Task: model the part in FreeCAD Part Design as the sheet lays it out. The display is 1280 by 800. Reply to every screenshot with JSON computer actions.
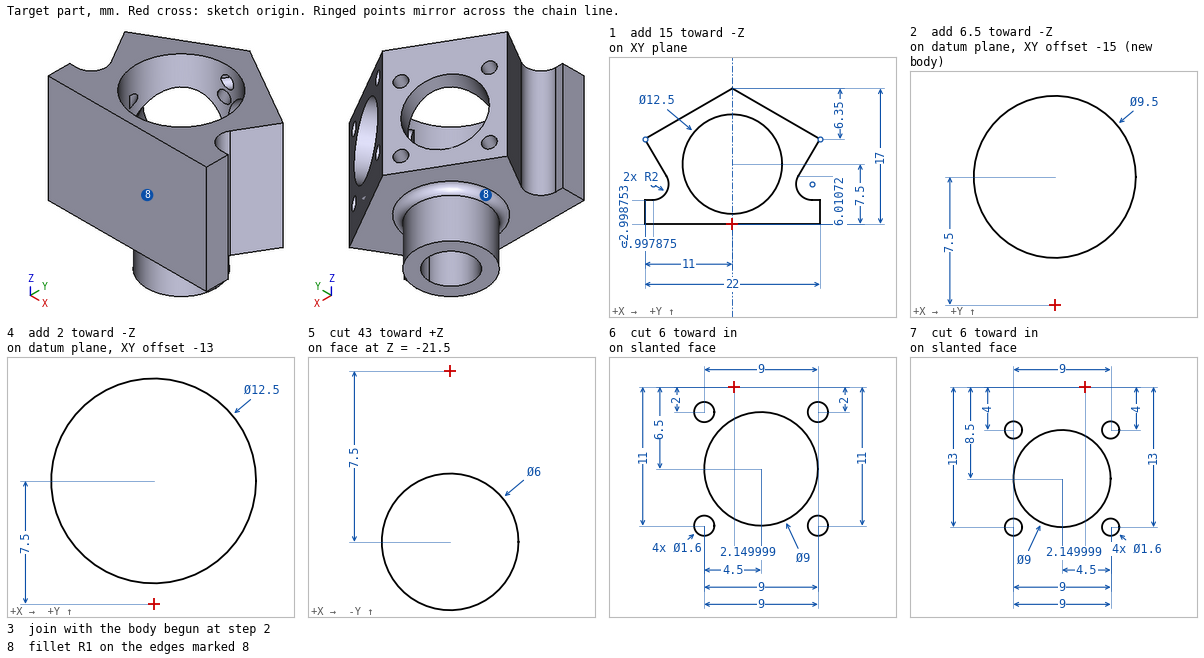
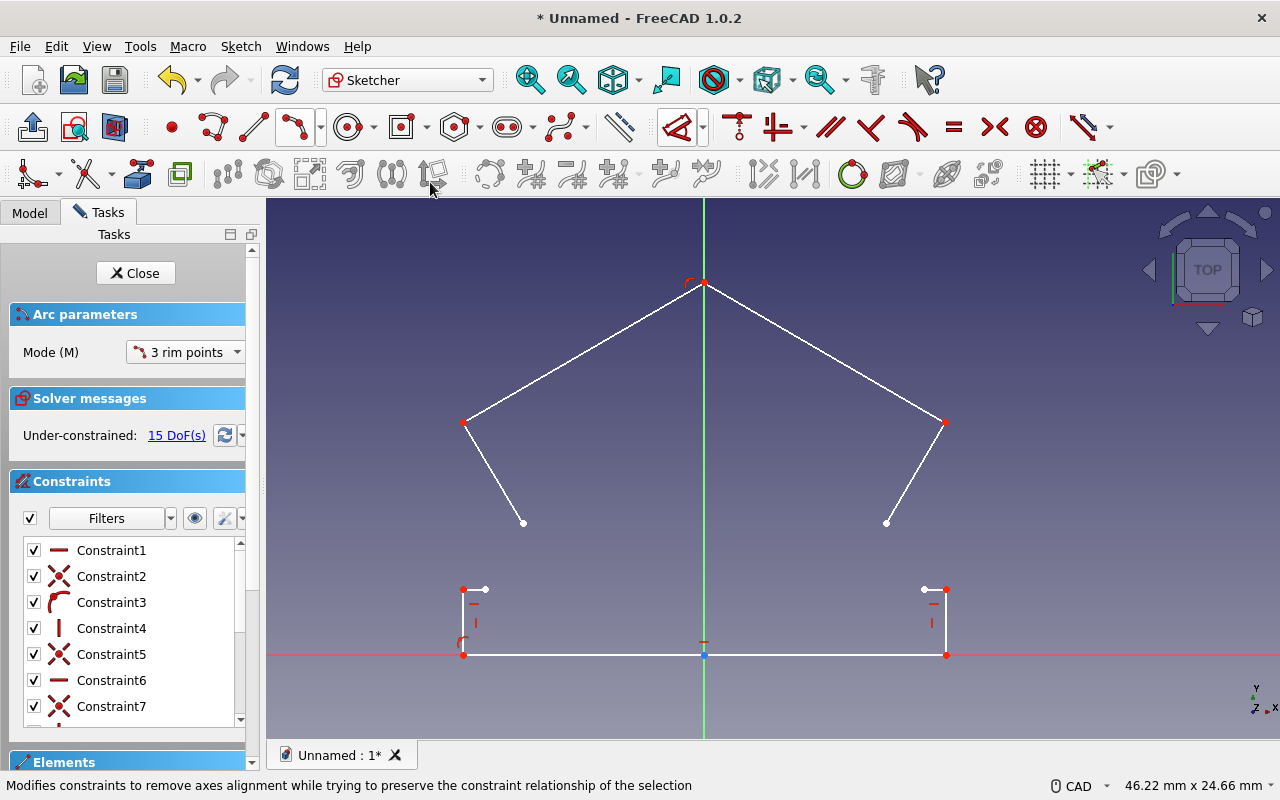
{"action": "scroll", "coordinate": [924, 589], "scroll_direction": "up", "scroll_amount": 2}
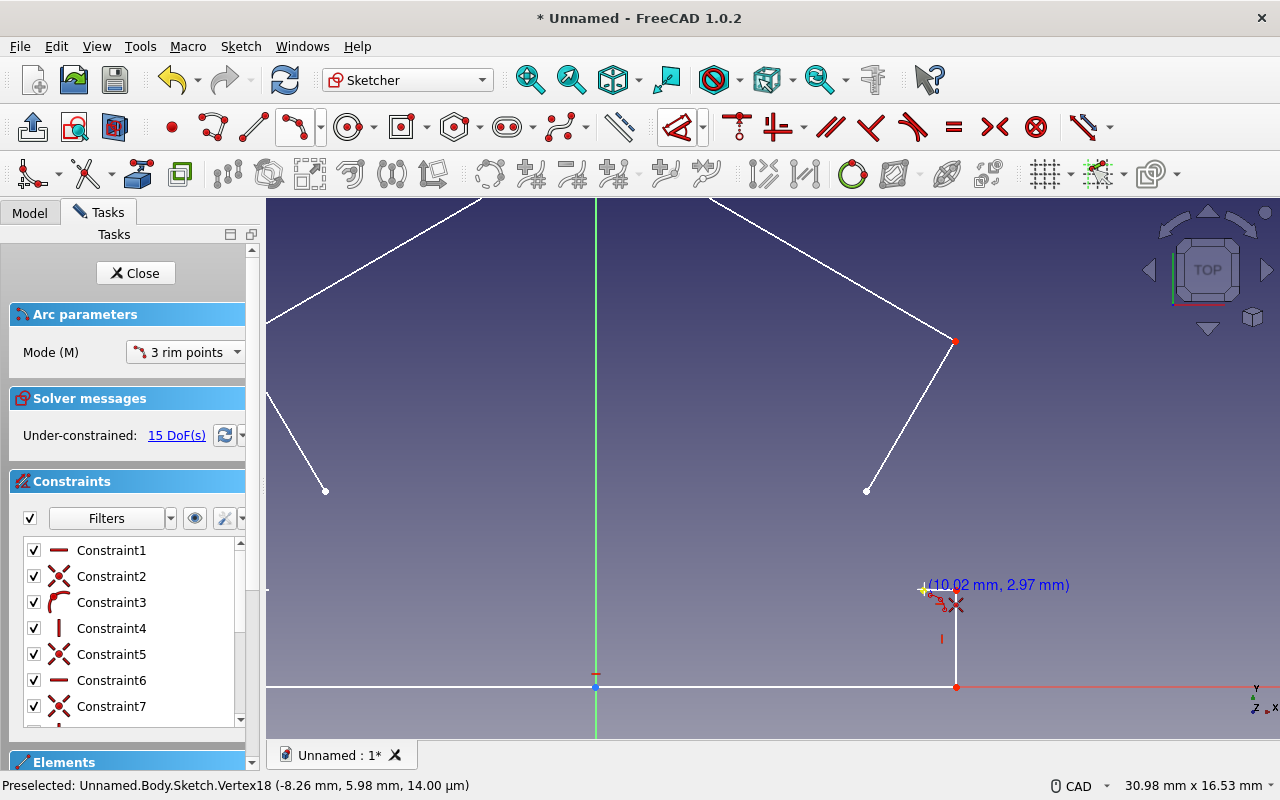
{"action": "left_click", "coordinate": [924, 590]}
{"action": "left_click", "coordinate": [867, 492]}
{"action": "left_click", "coordinate": [866, 556]}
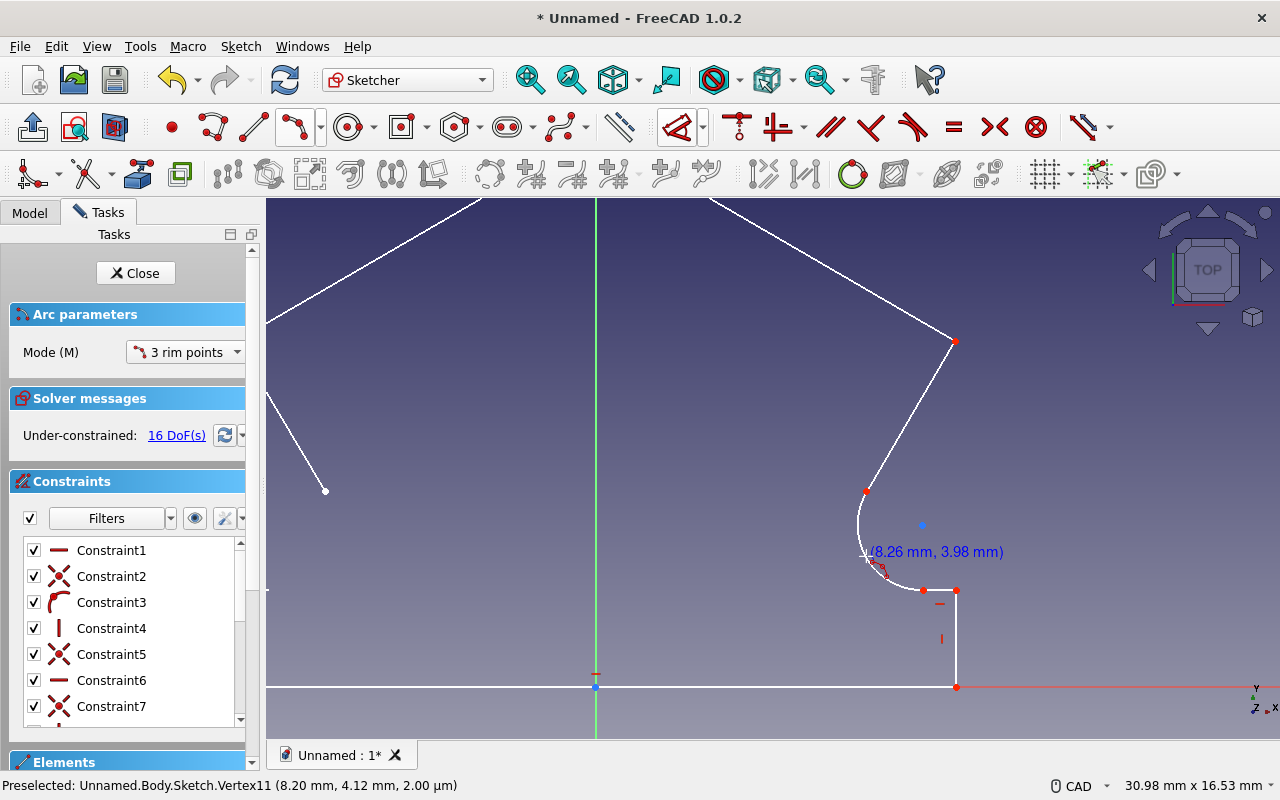
{"action": "left_click", "coordinate": [325, 492]}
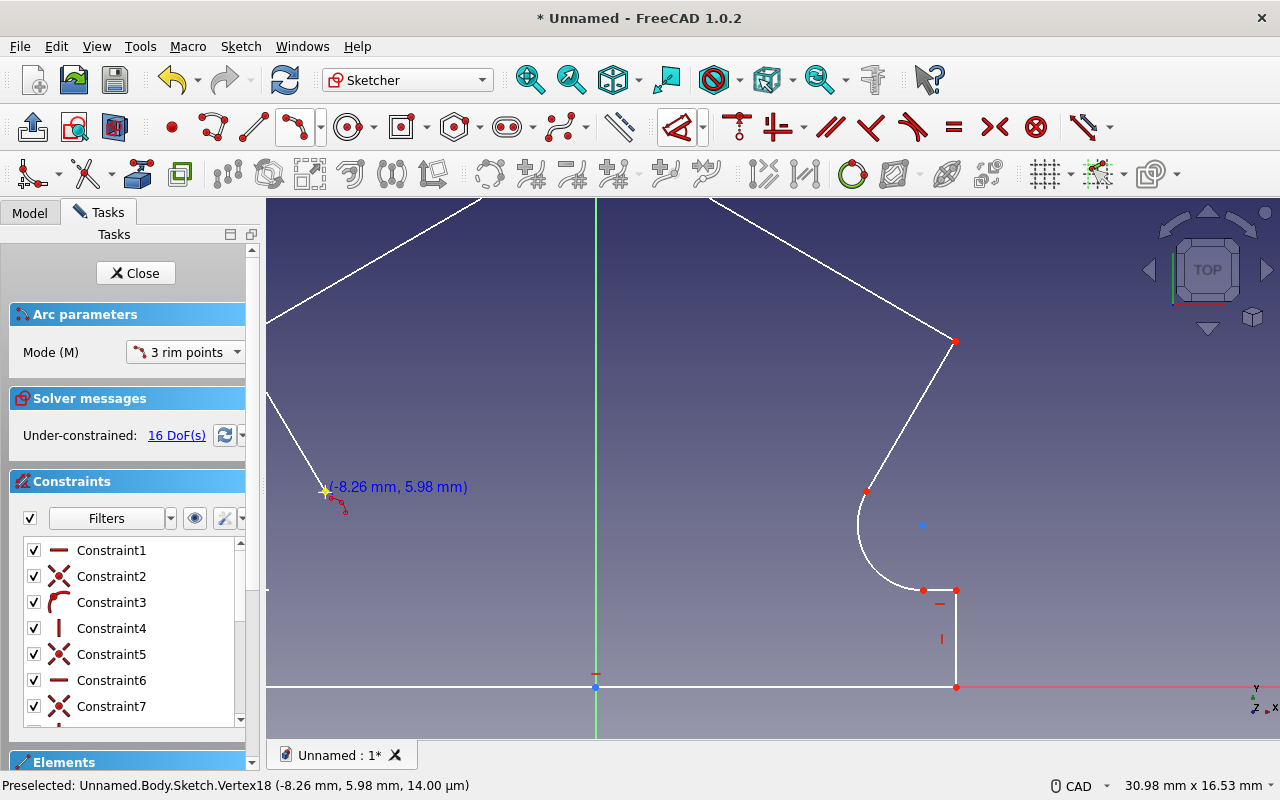
{"action": "scroll", "coordinate": [926, 589], "scroll_direction": "down", "scroll_amount": 2}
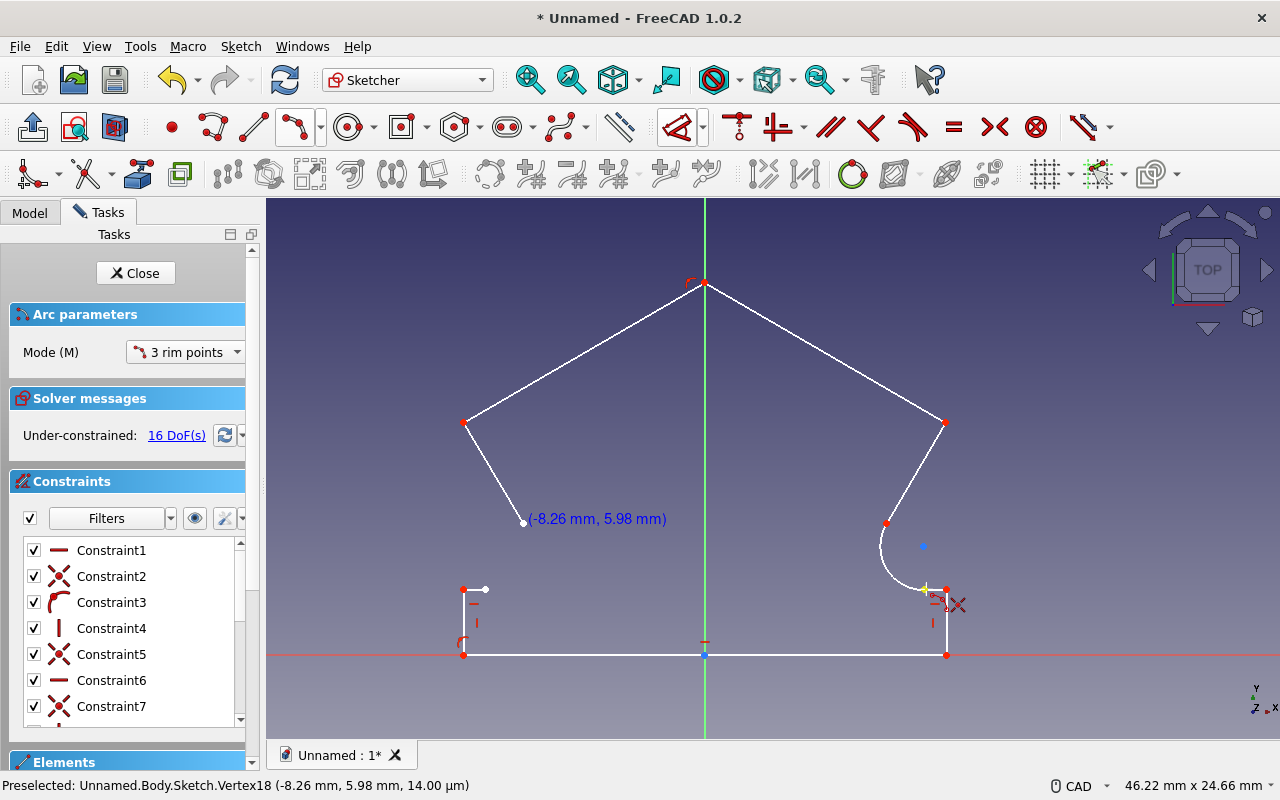
{"action": "scroll", "coordinate": [485, 589], "scroll_direction": "up", "scroll_amount": 2}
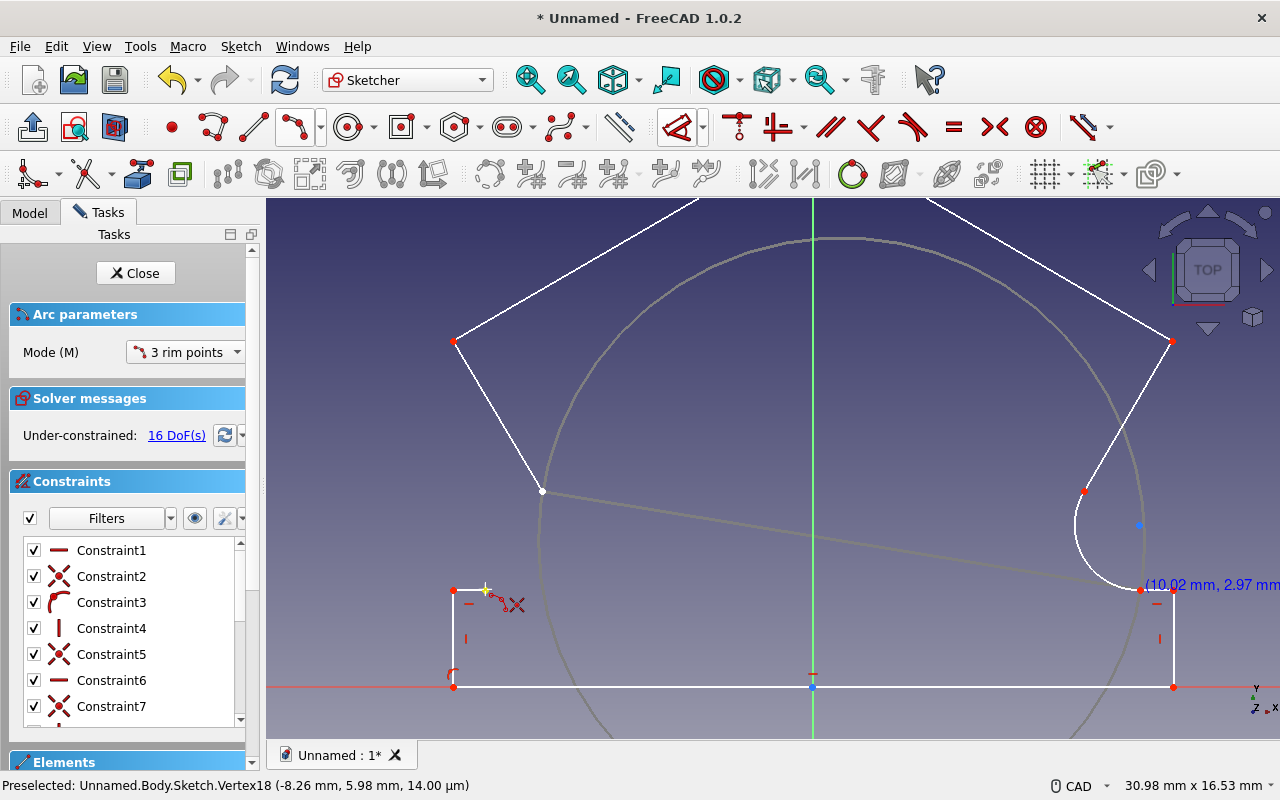
{"action": "left_click", "coordinate": [486, 590]}
{"action": "left_click", "coordinate": [542, 556]}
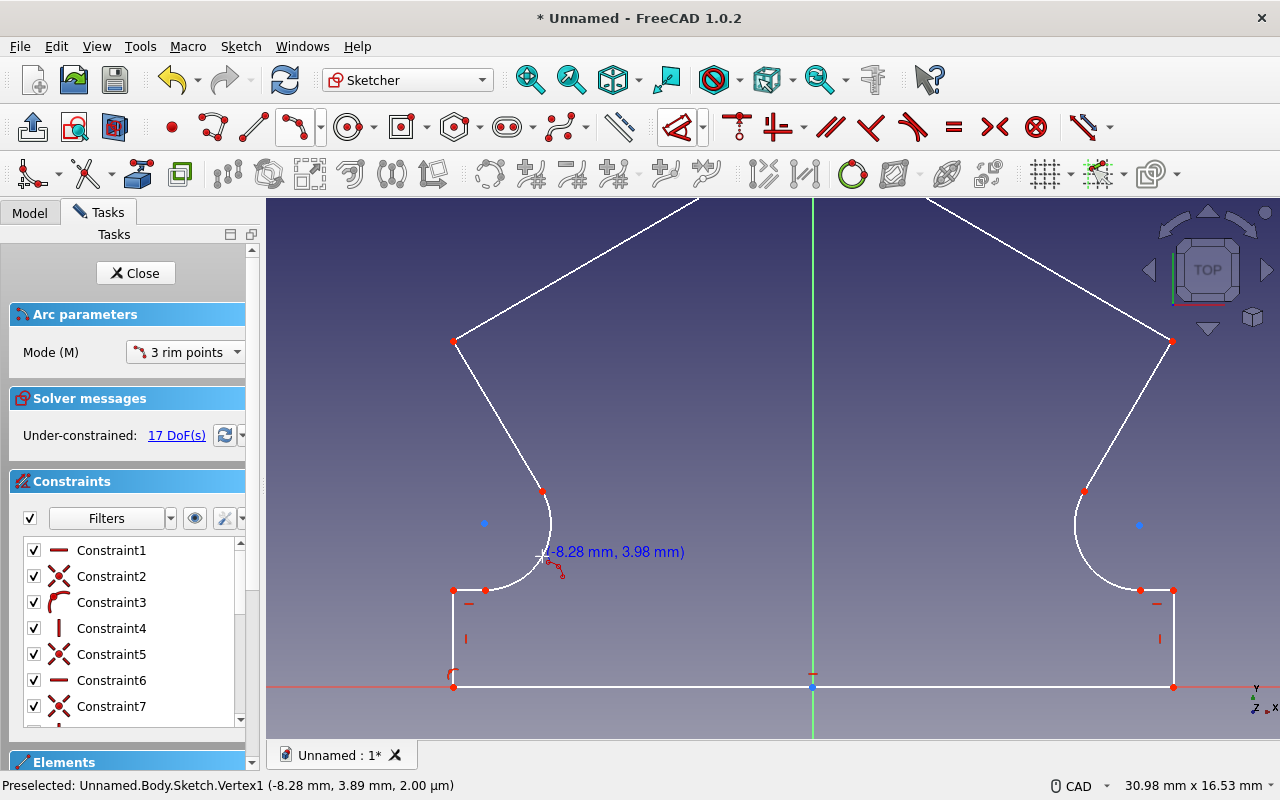
{"action": "left_click", "coordinate": [348, 128]}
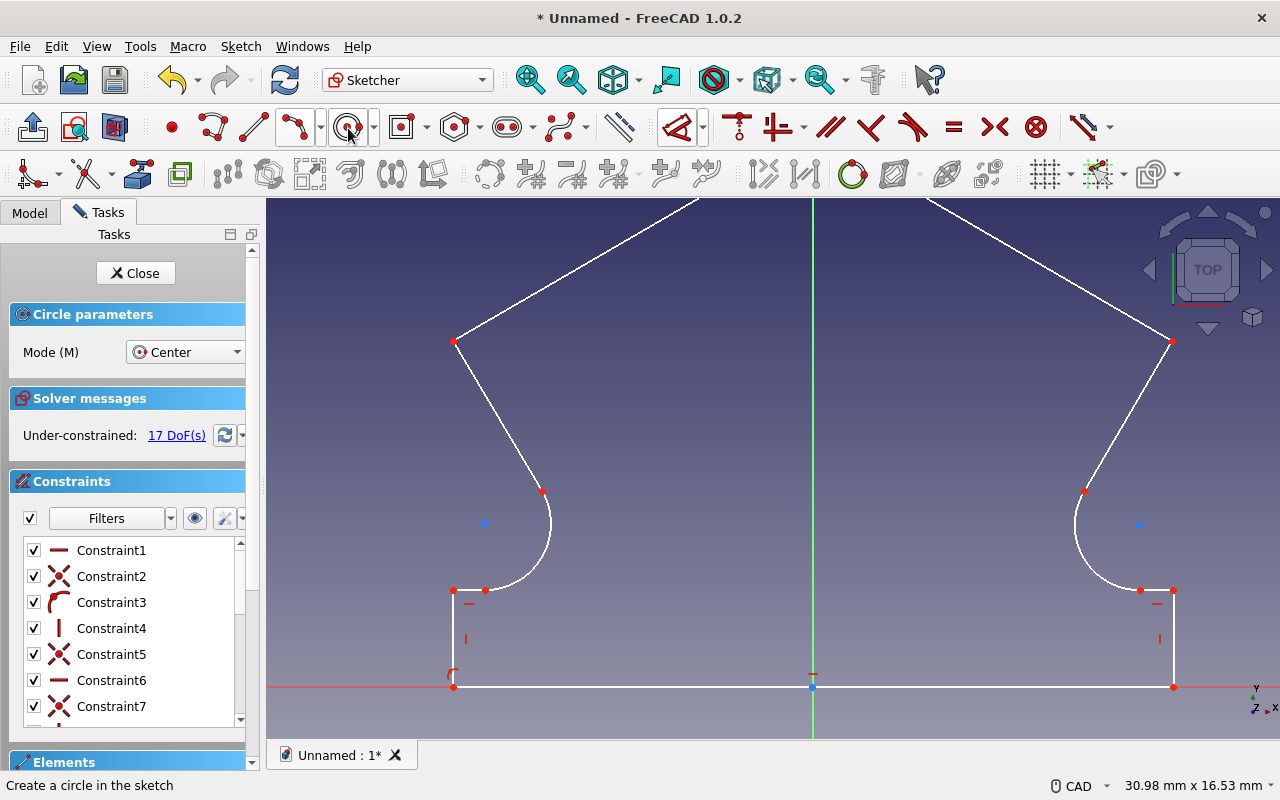
{"action": "left_click", "coordinate": [813, 442]}
{"action": "mouse_move", "coordinate": [958, 297]}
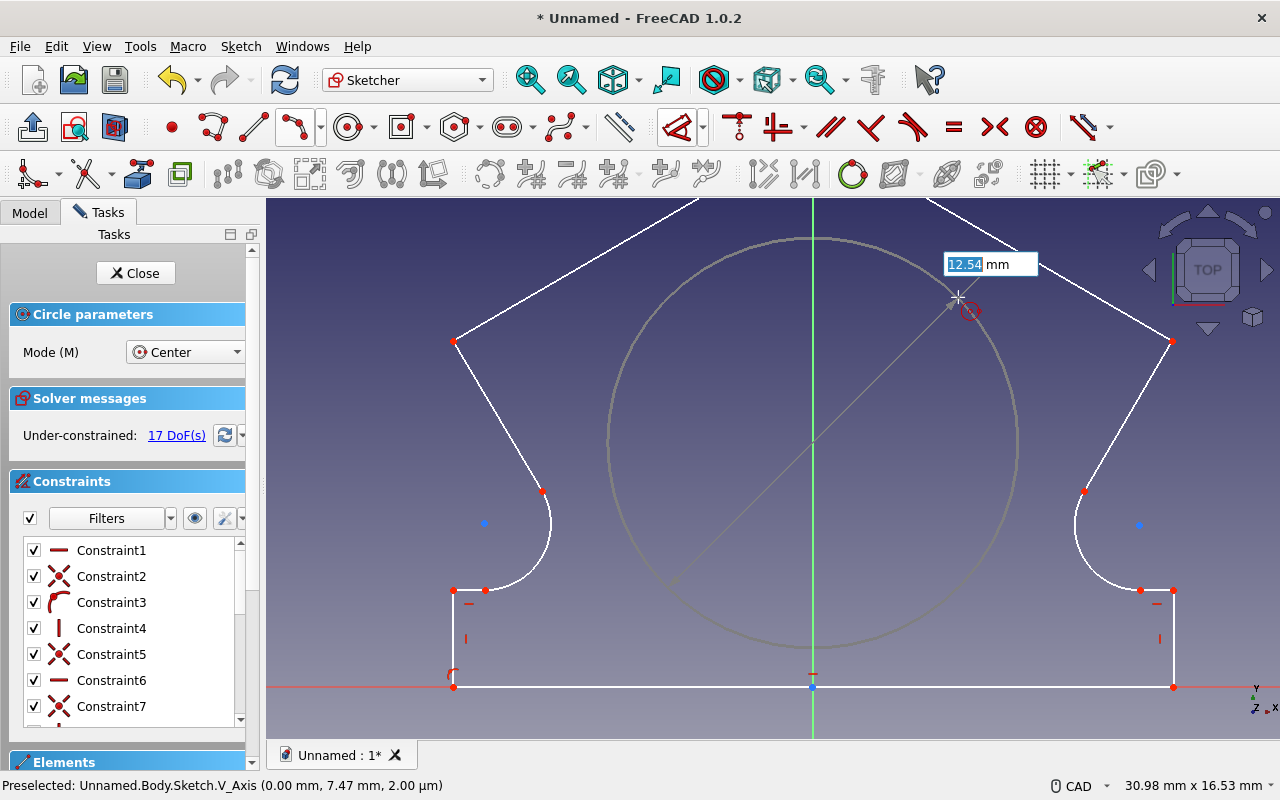
{"action": "type", "text": "12.5"}
{"action": "key", "text": "Return"}
{"action": "key", "text": "Escape"}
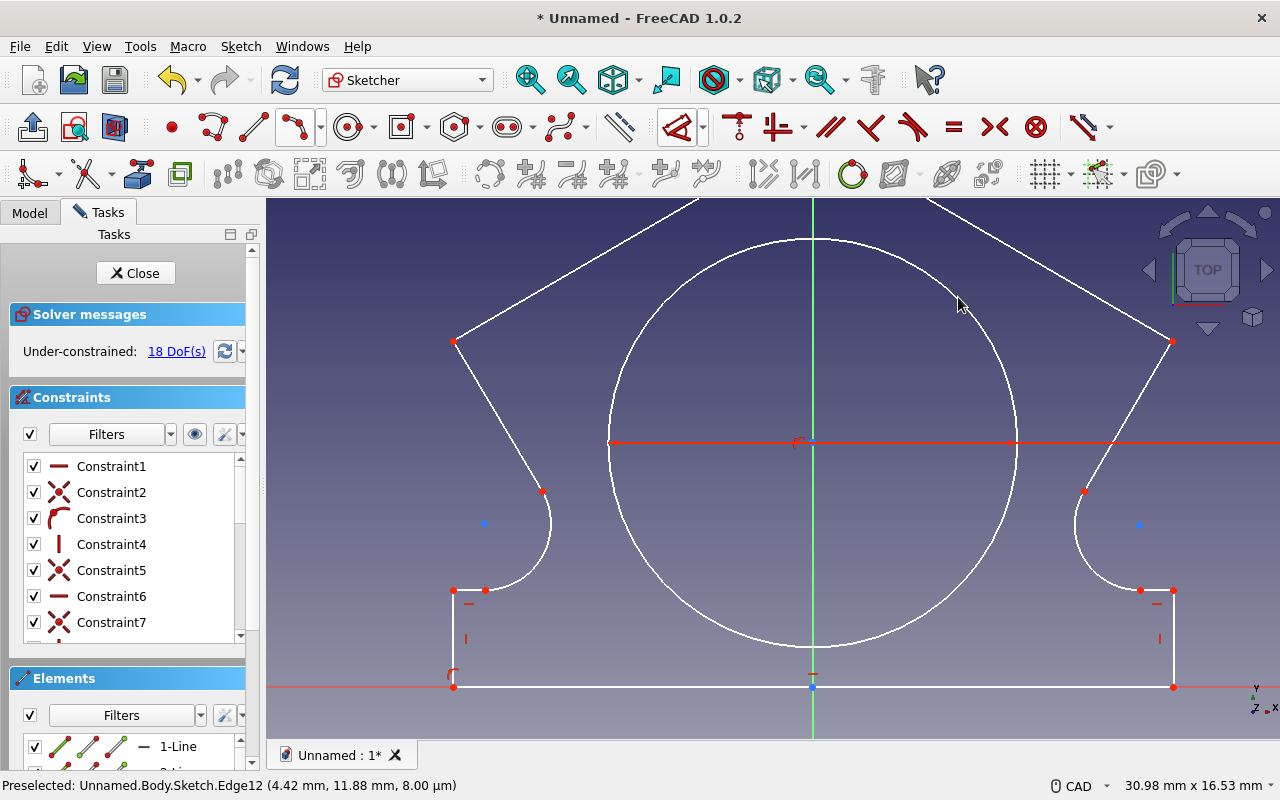
{"action": "scroll", "coordinate": [476, 590], "scroll_direction": "up", "scroll_amount": 2}